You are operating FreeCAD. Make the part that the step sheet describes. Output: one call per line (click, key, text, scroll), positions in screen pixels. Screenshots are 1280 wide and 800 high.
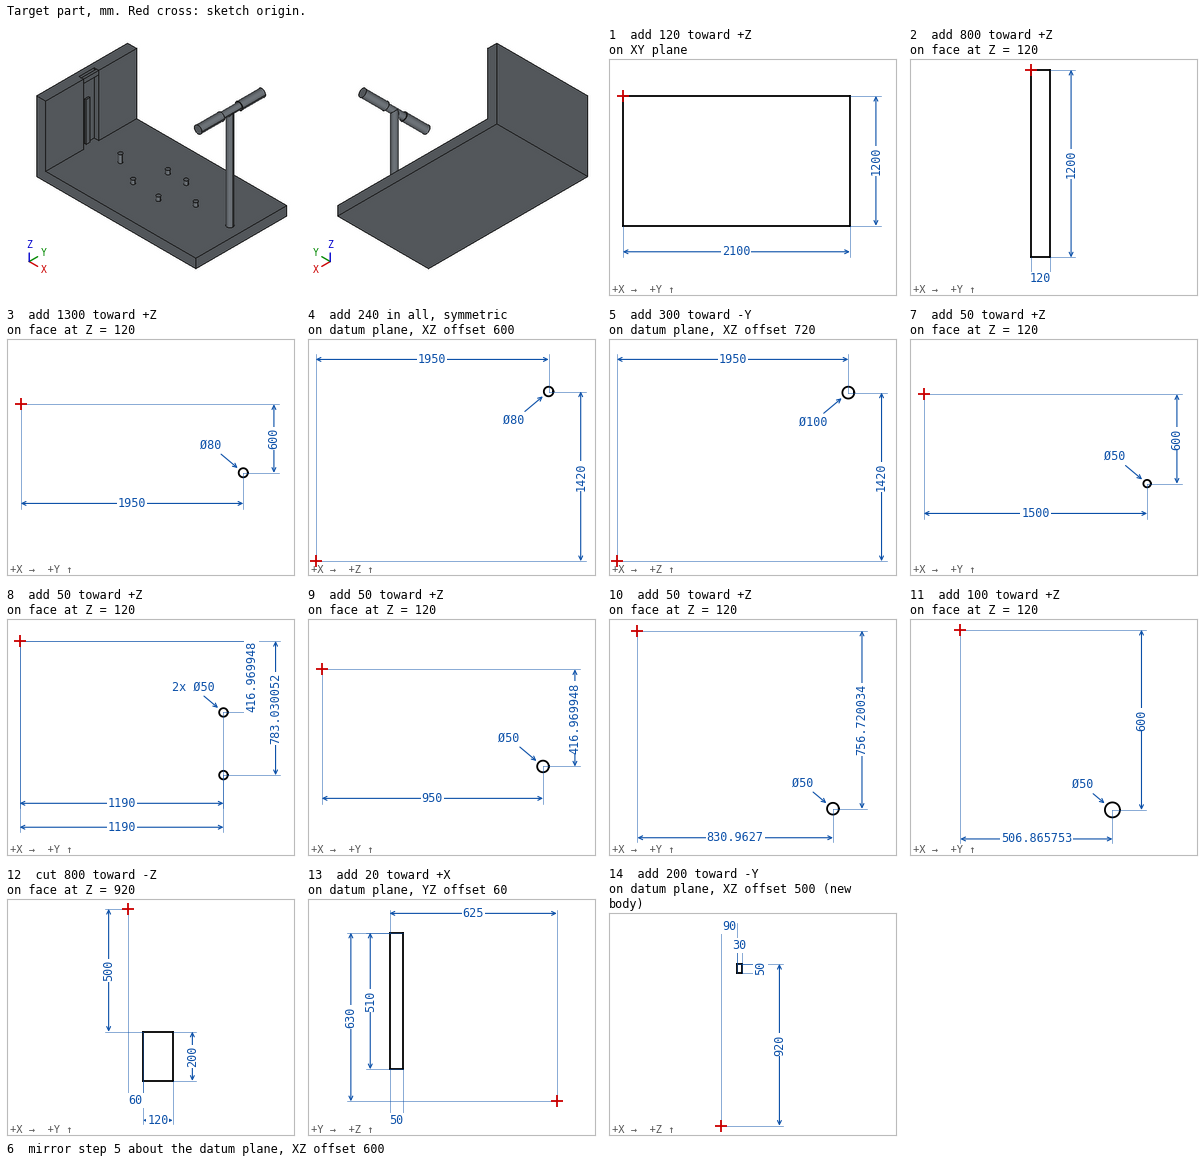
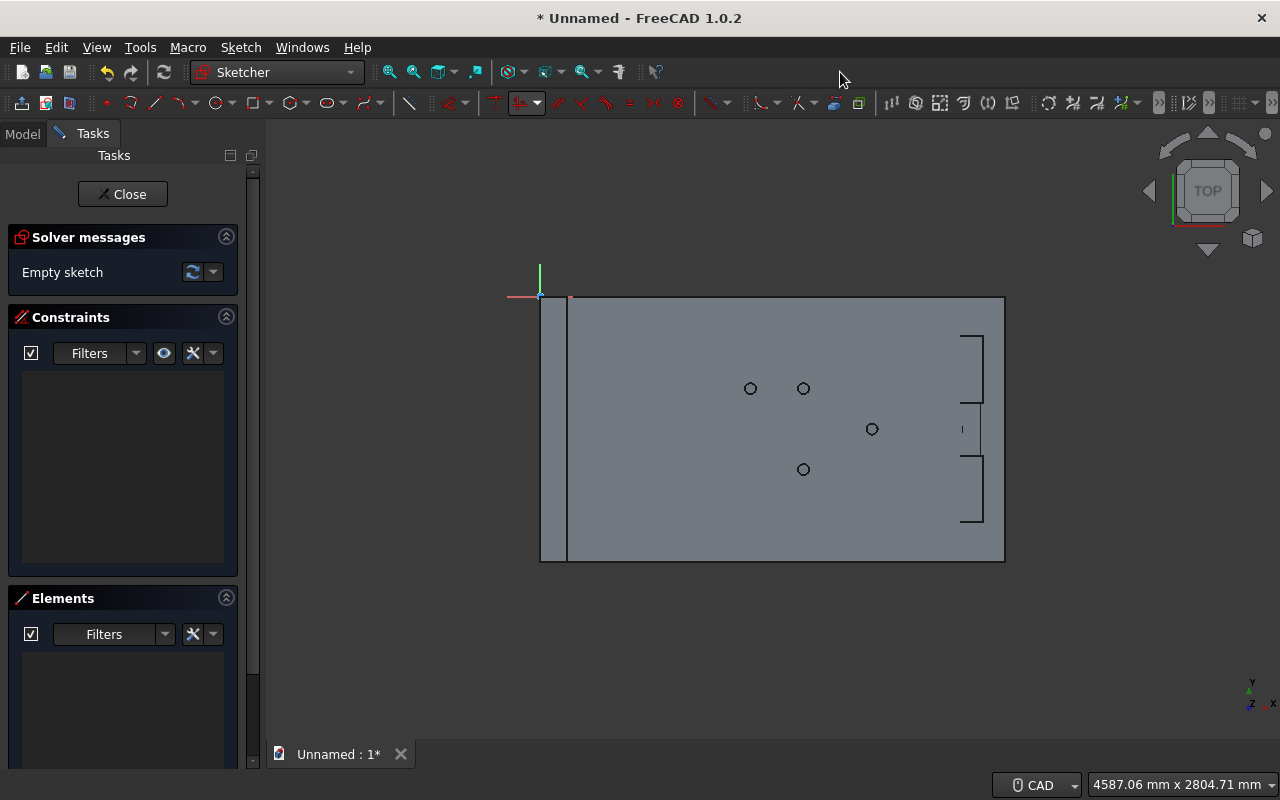
scroll(725, 466, up, 15)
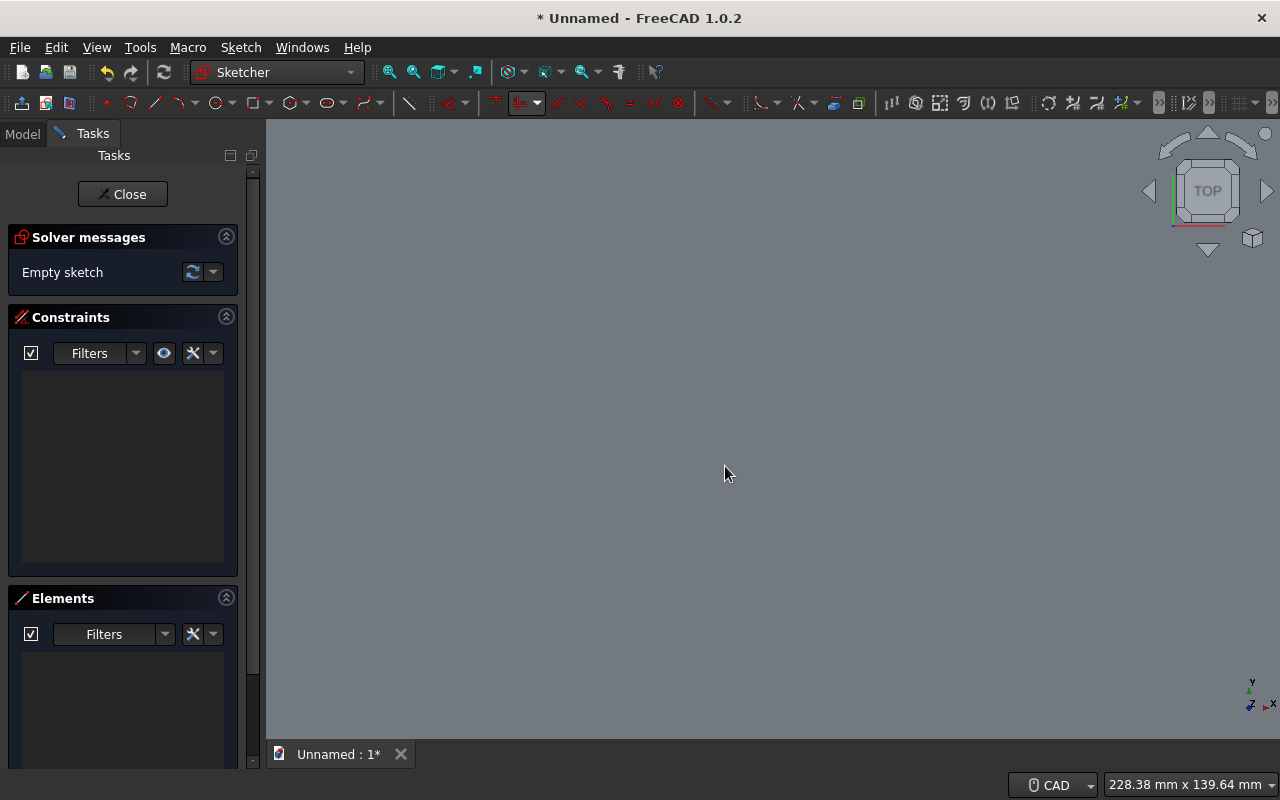
scroll(693, 390, up, 3)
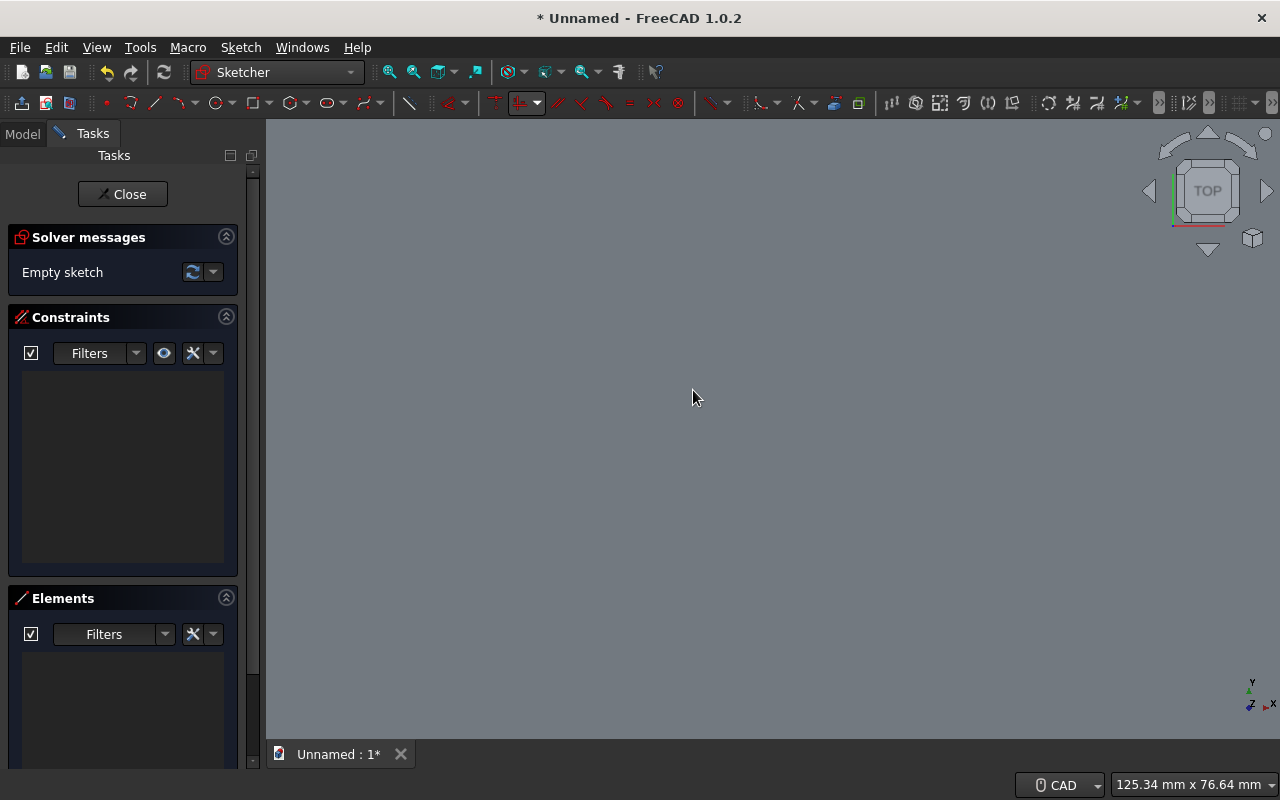
click(216, 104)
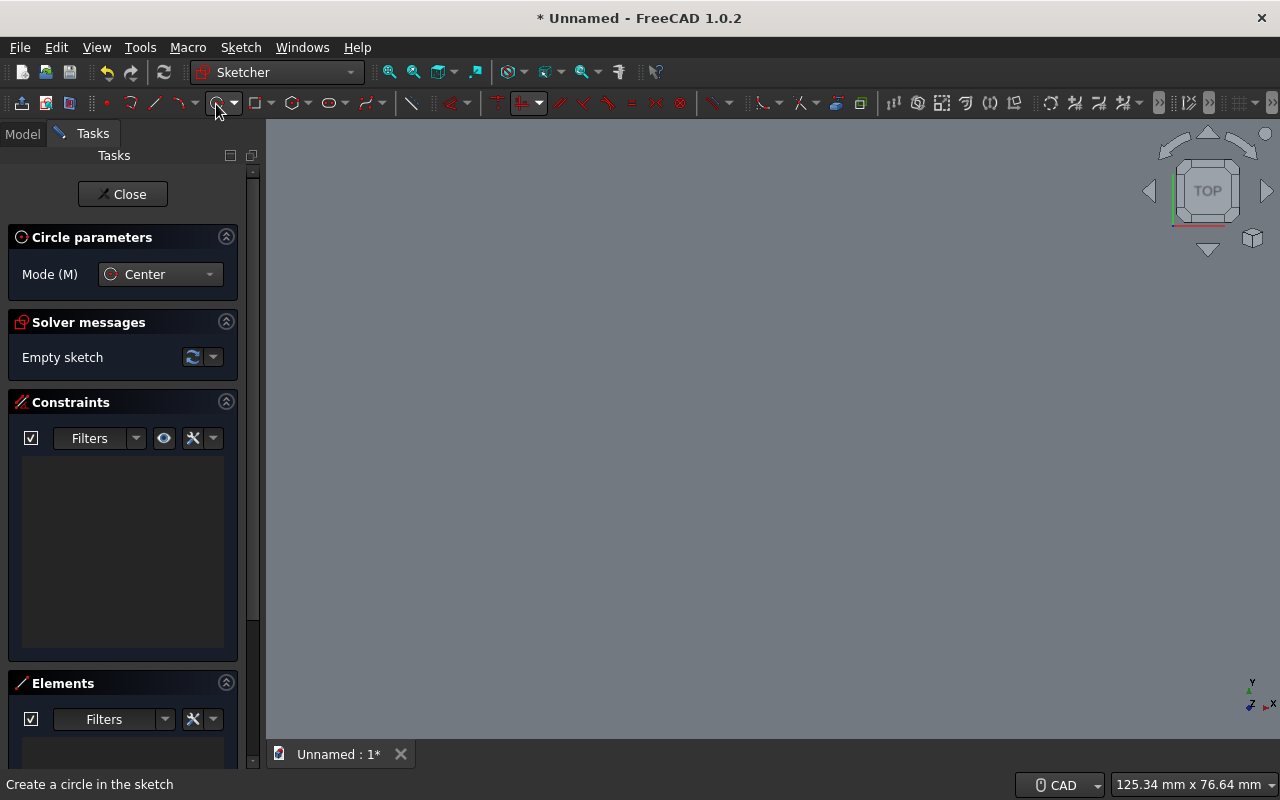
click(704, 429)
move(847, 286)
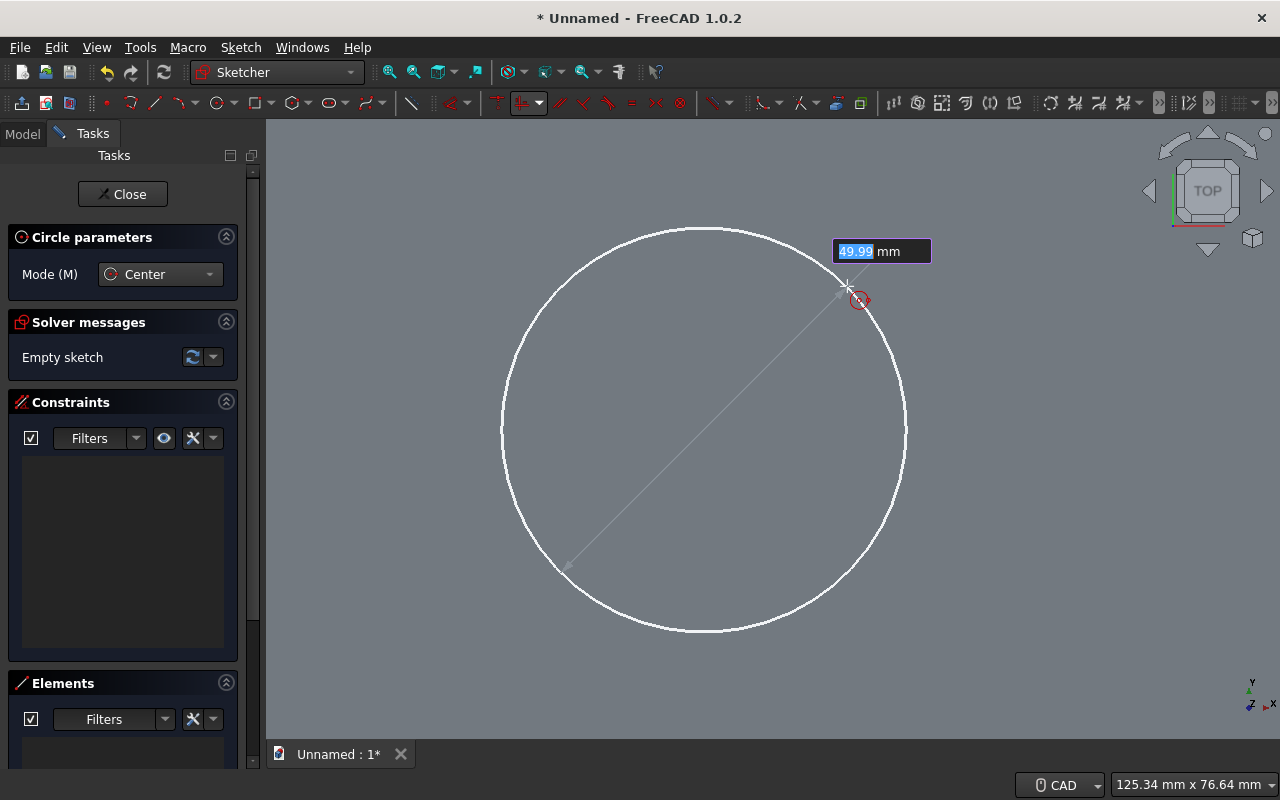
text(50)
key(Return)
key(Escape)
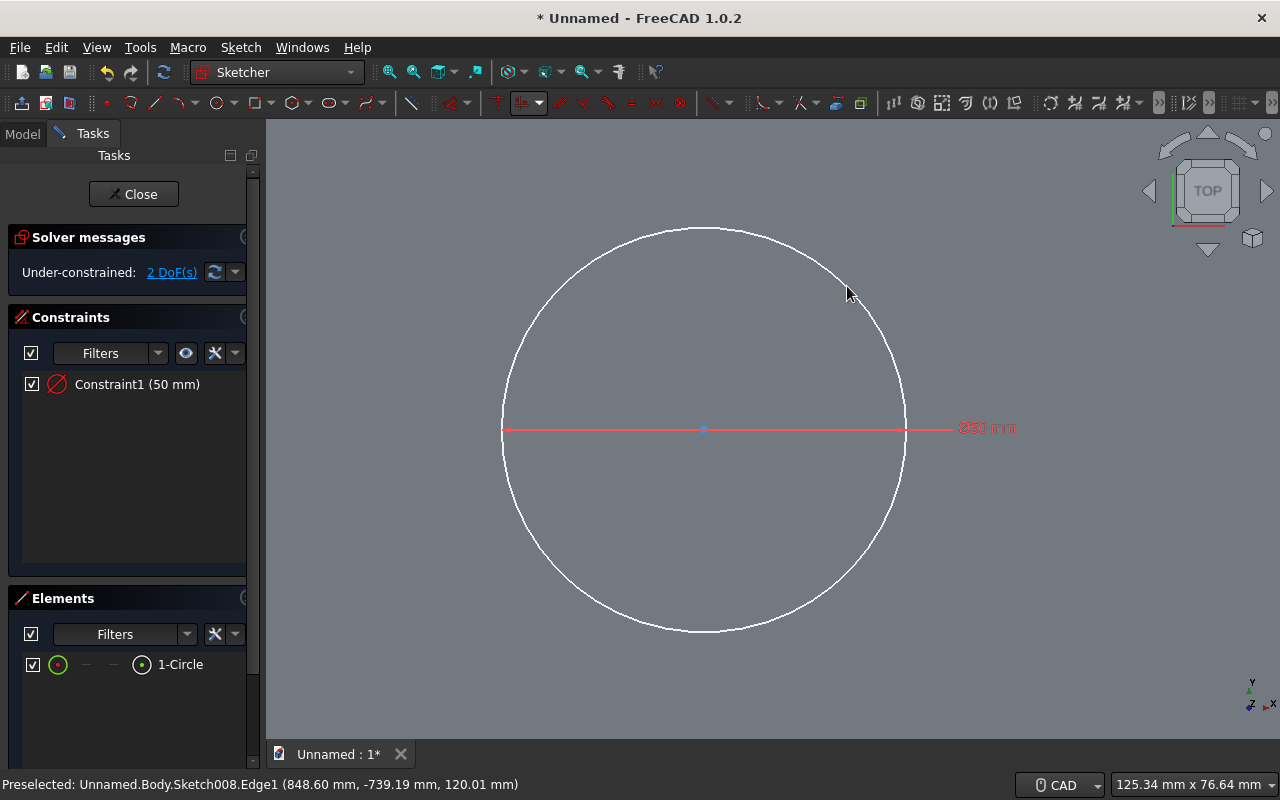
key(d)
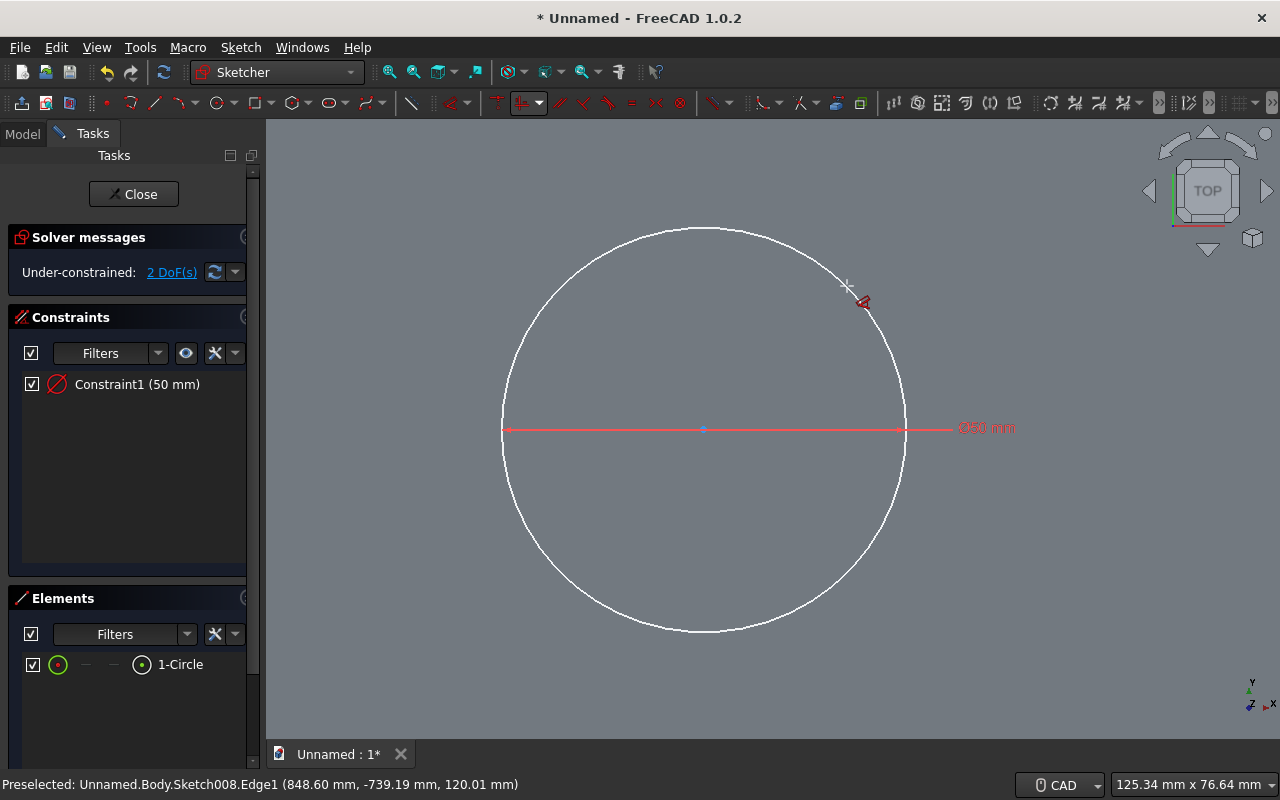
click(704, 430)
click(405, 464)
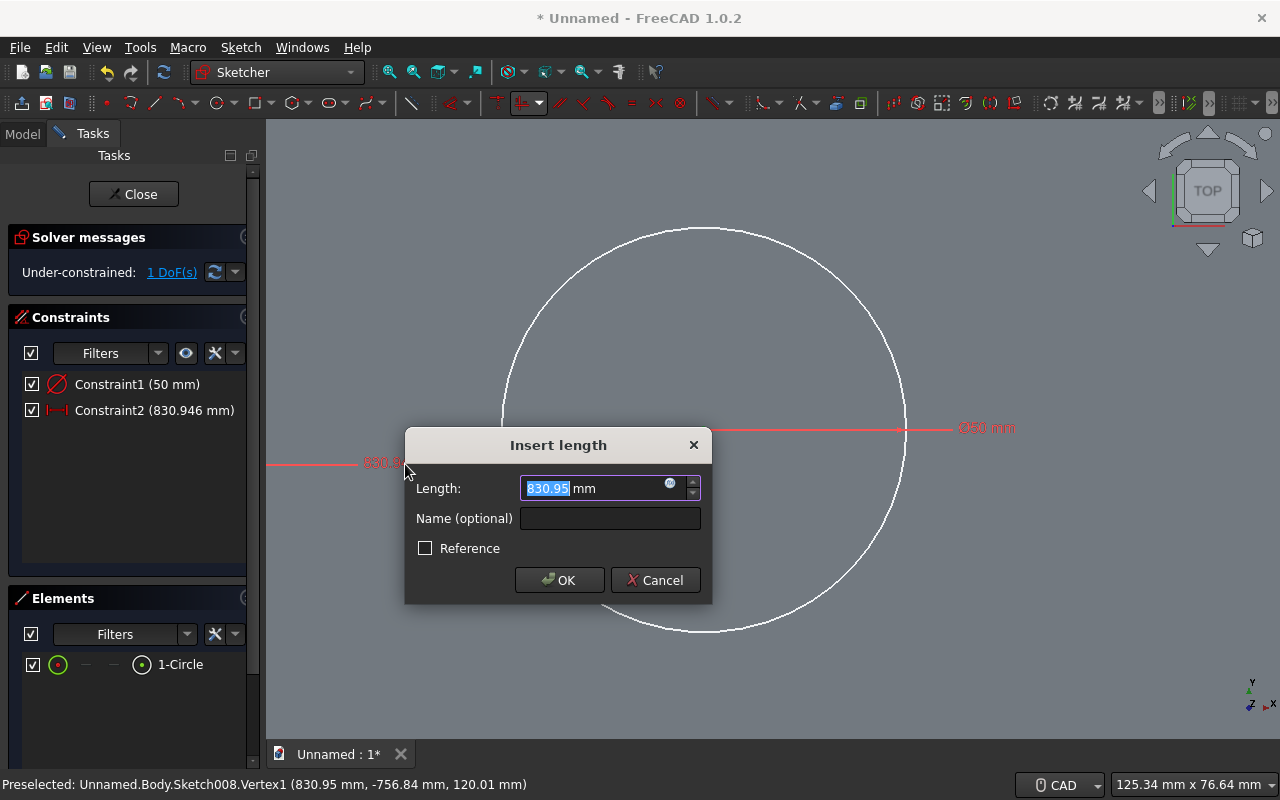
text(830.9627)
key(Return)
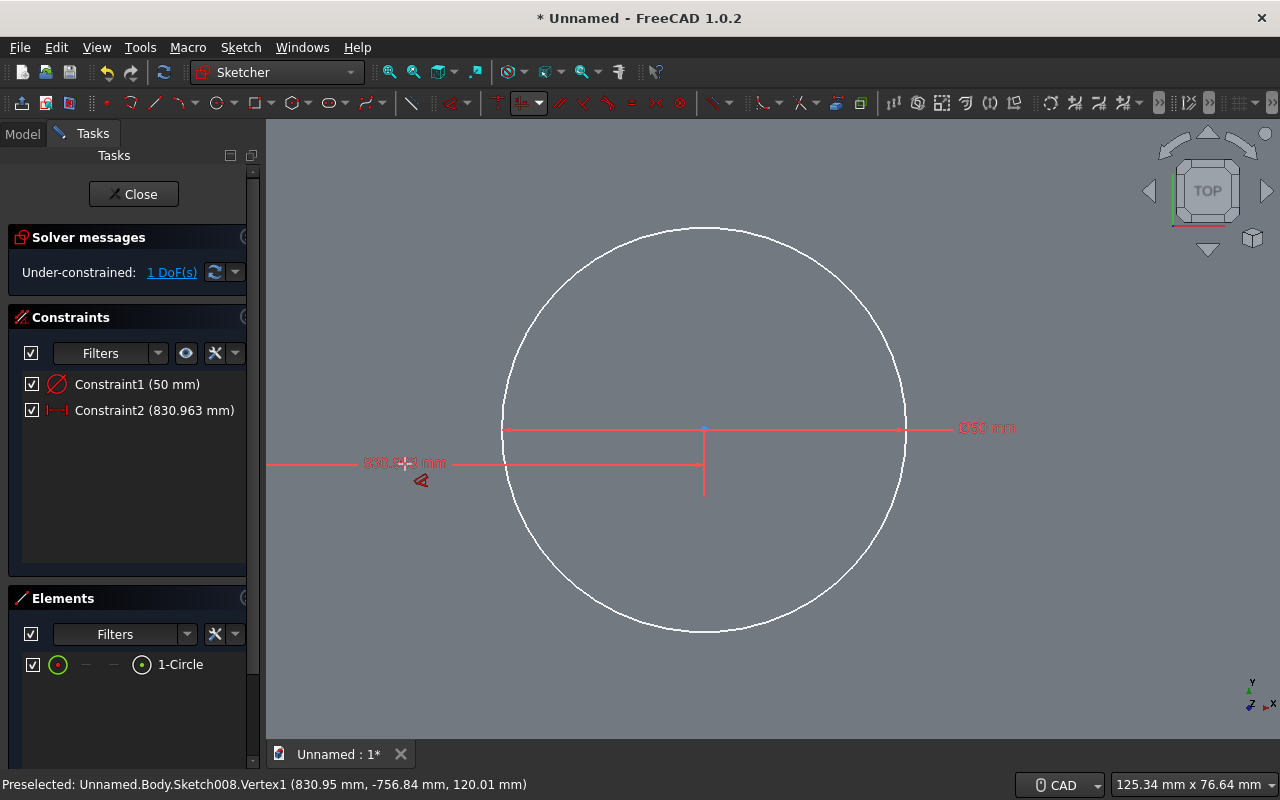
click(704, 430)
click(738, 288)